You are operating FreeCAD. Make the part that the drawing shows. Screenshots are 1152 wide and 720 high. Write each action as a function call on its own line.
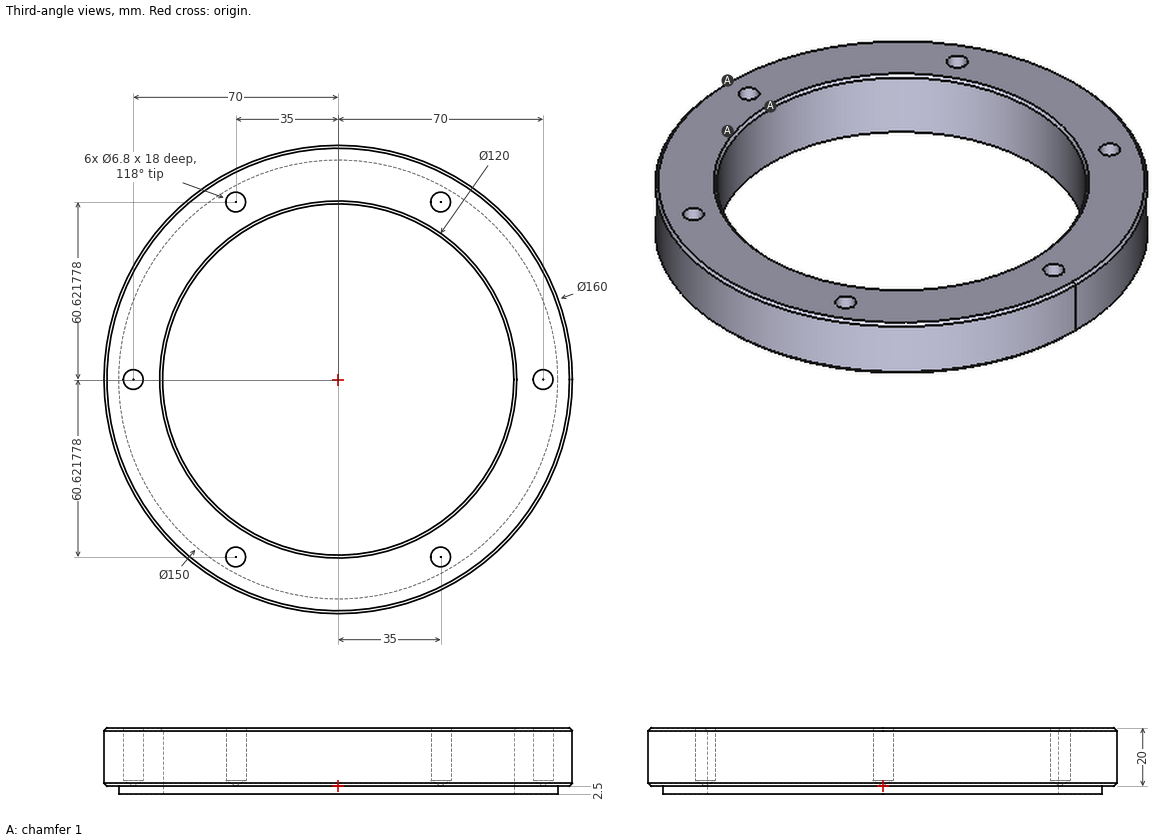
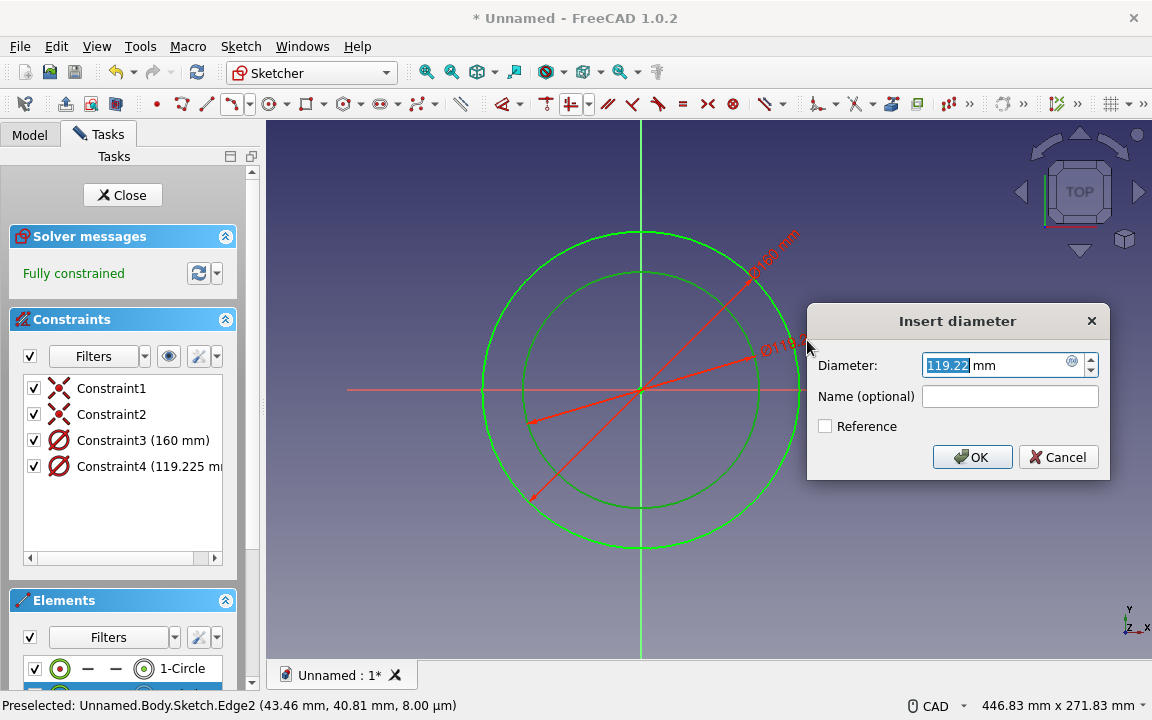
text(120)
key(Return)
key(Escape)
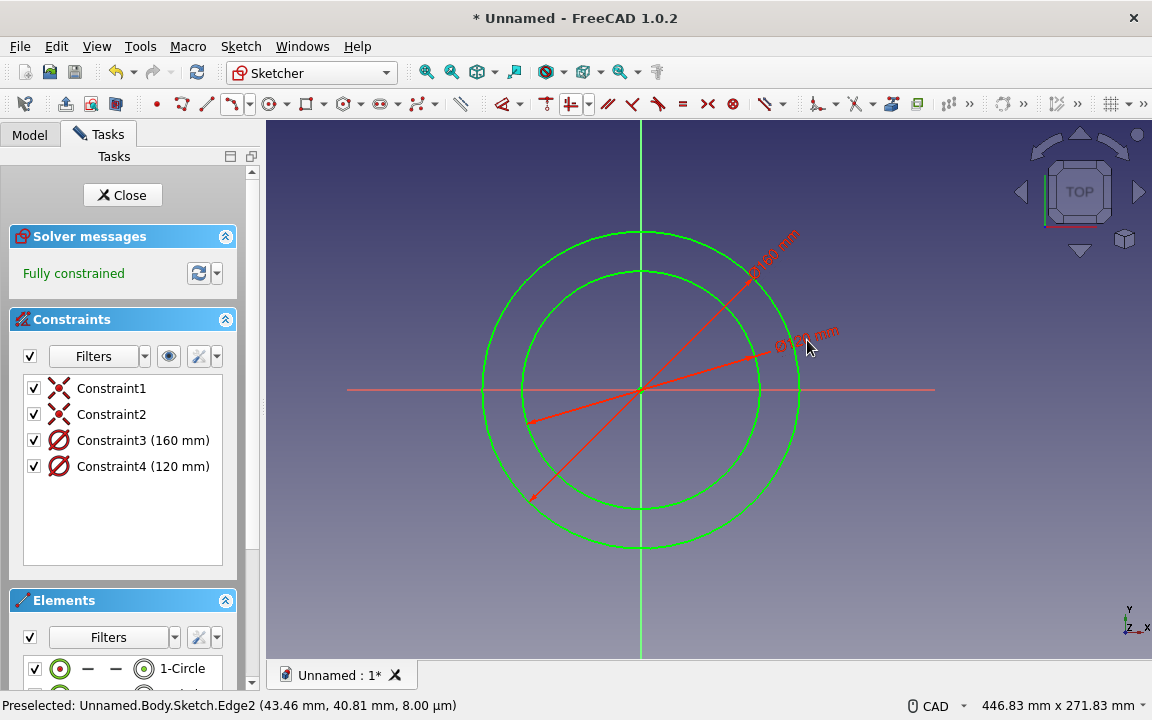
click(123, 195)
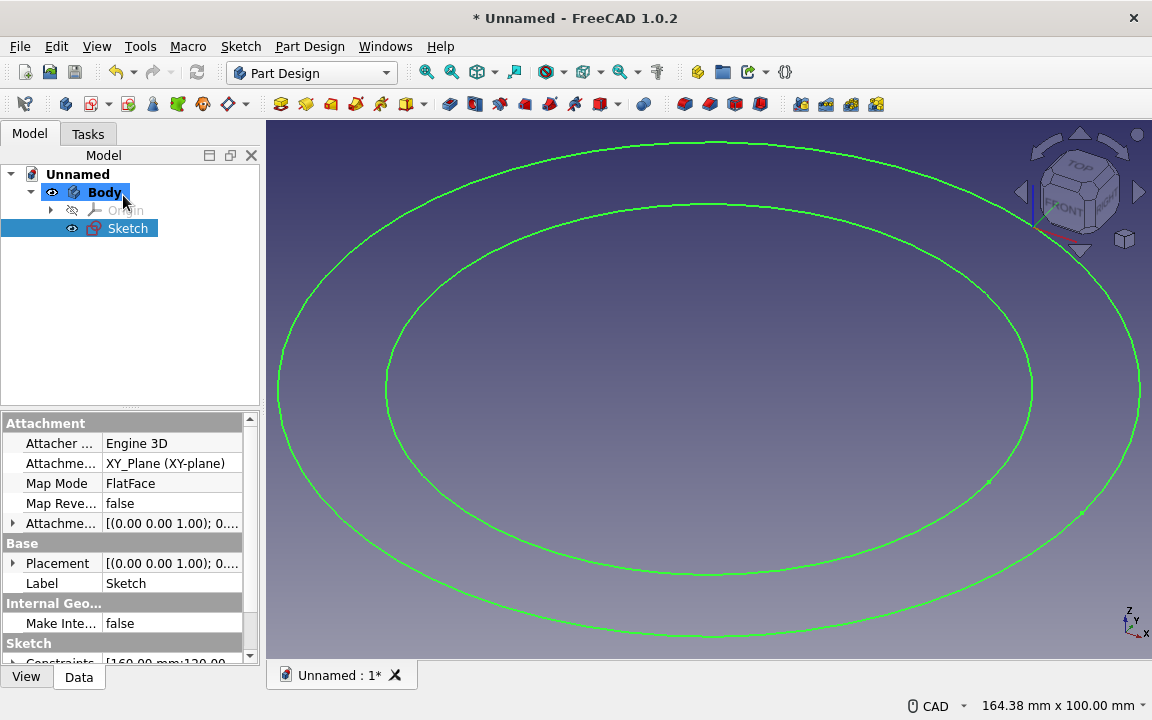
click(281, 104)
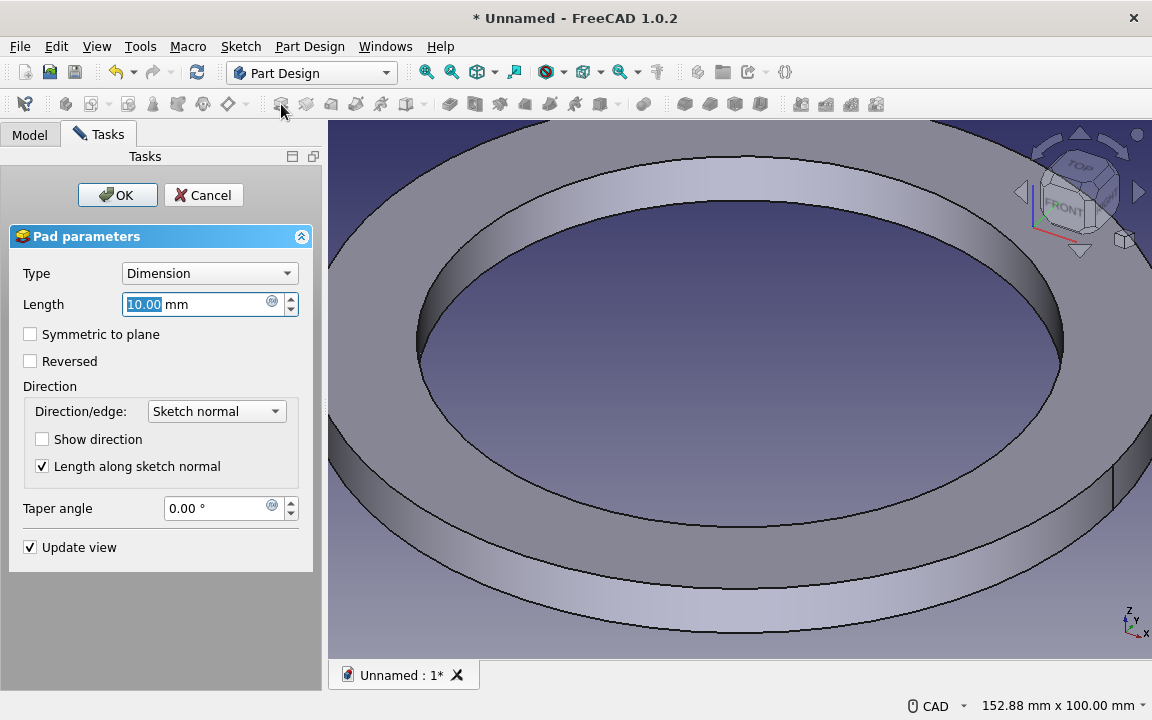
text(20)
key(Tab)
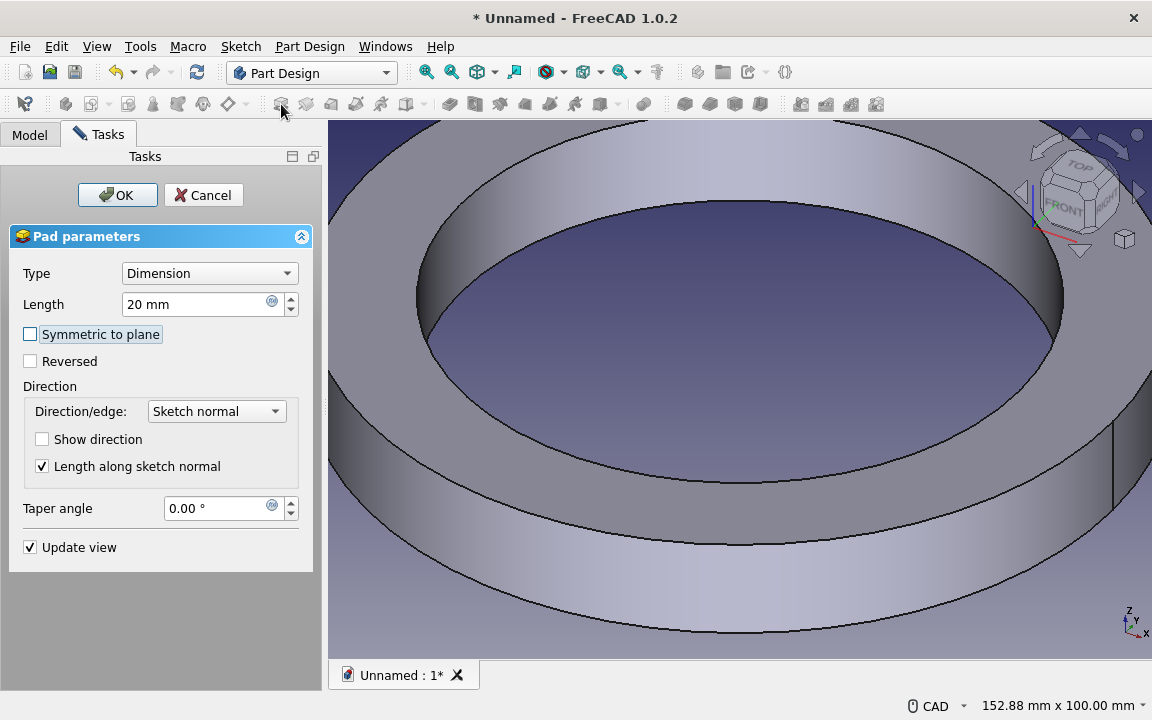
click(118, 195)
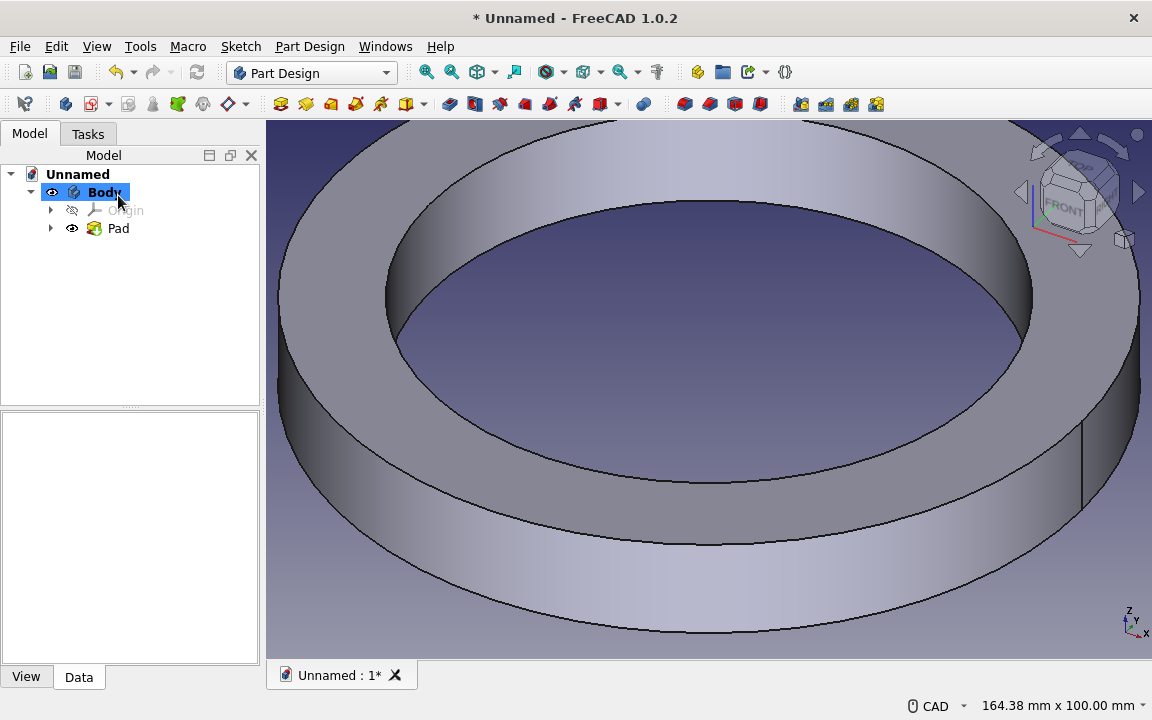
click(427, 72)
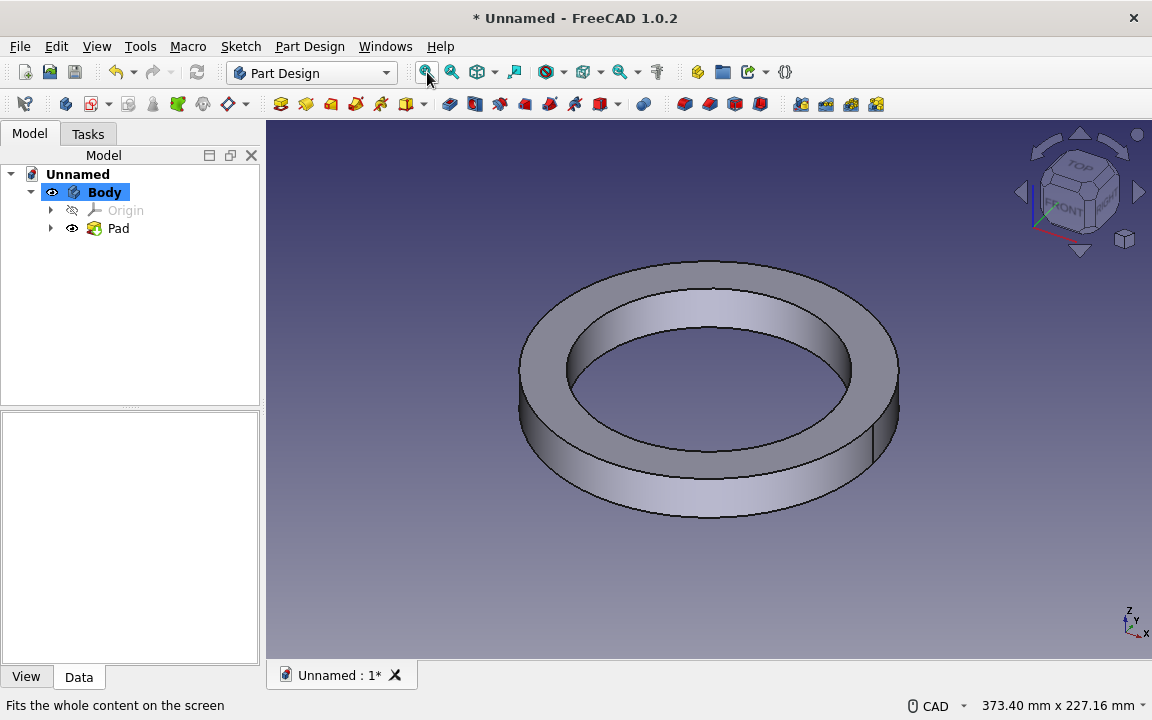
click(850, 416)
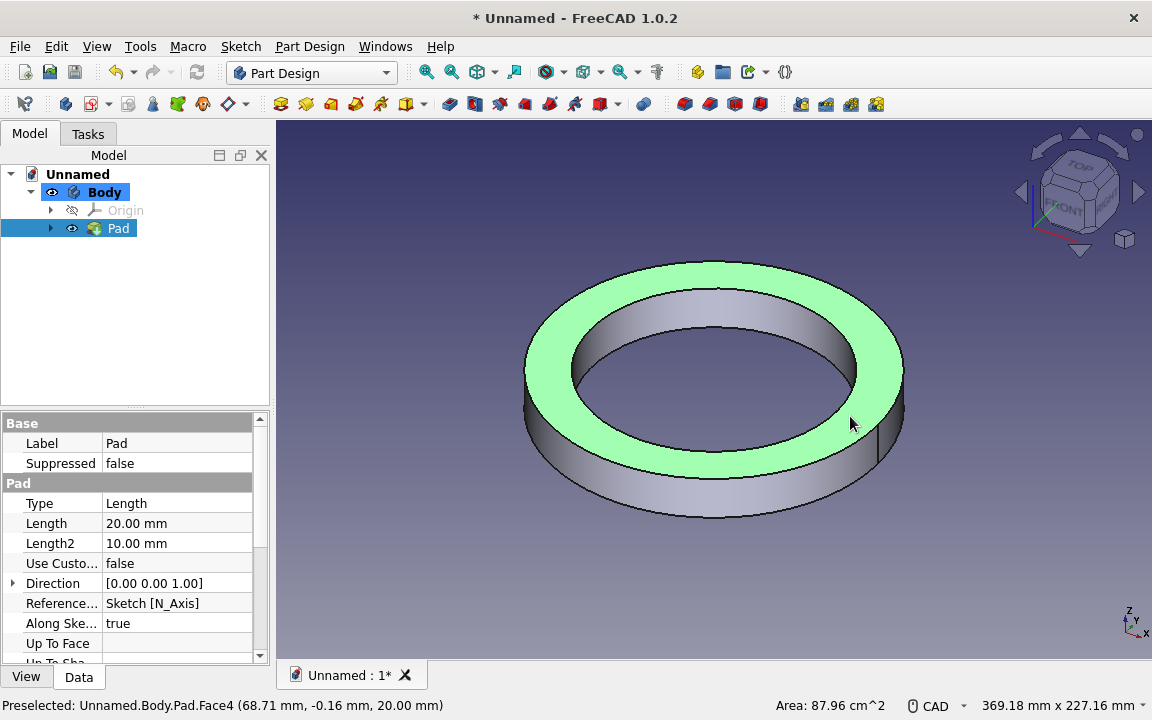
click(90, 104)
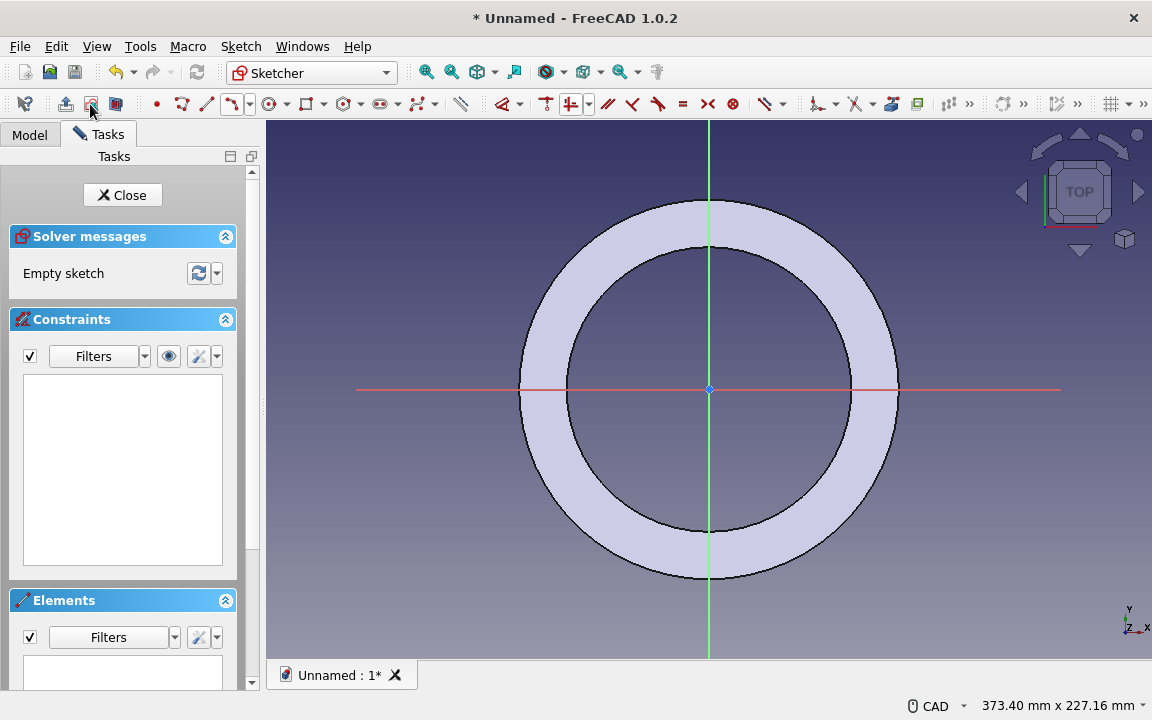
click(268, 104)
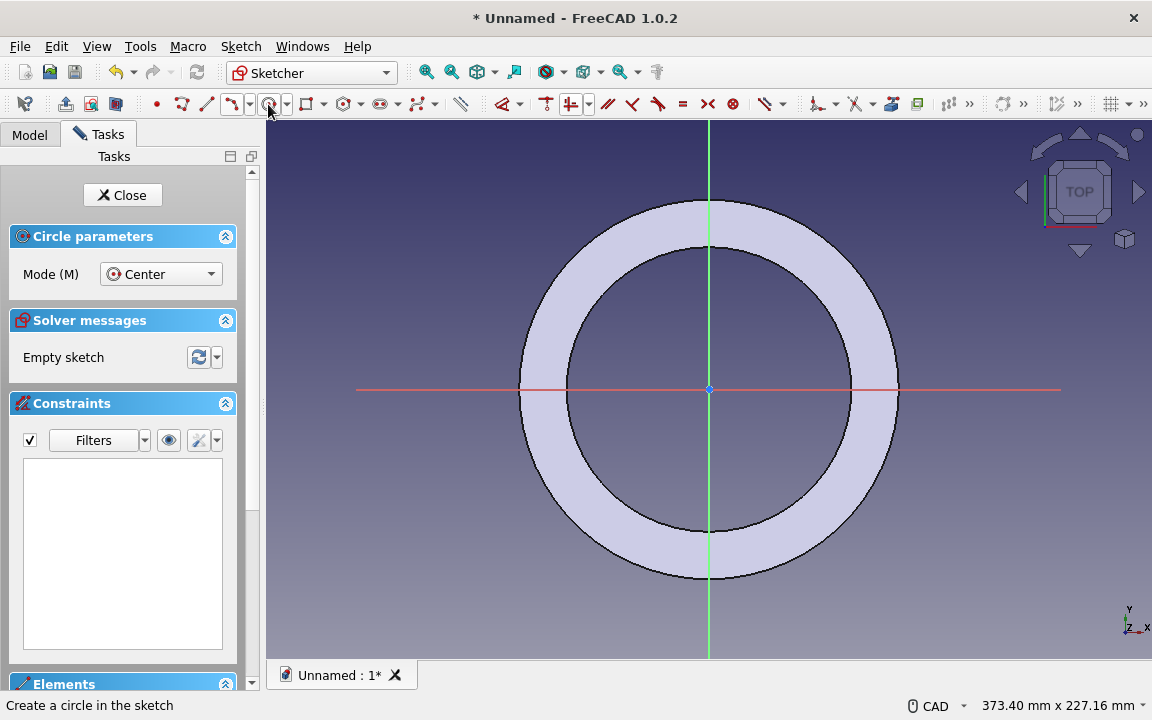
scroll(626, 246, up, 6)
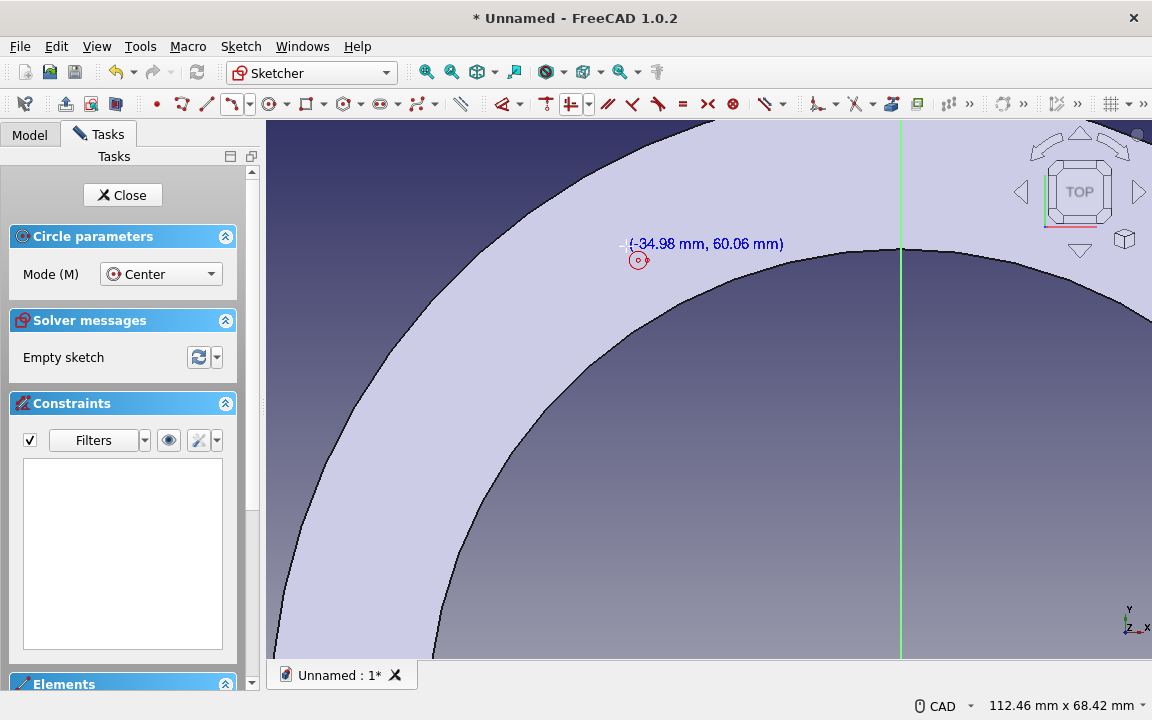
click(625, 244)
click(644, 225)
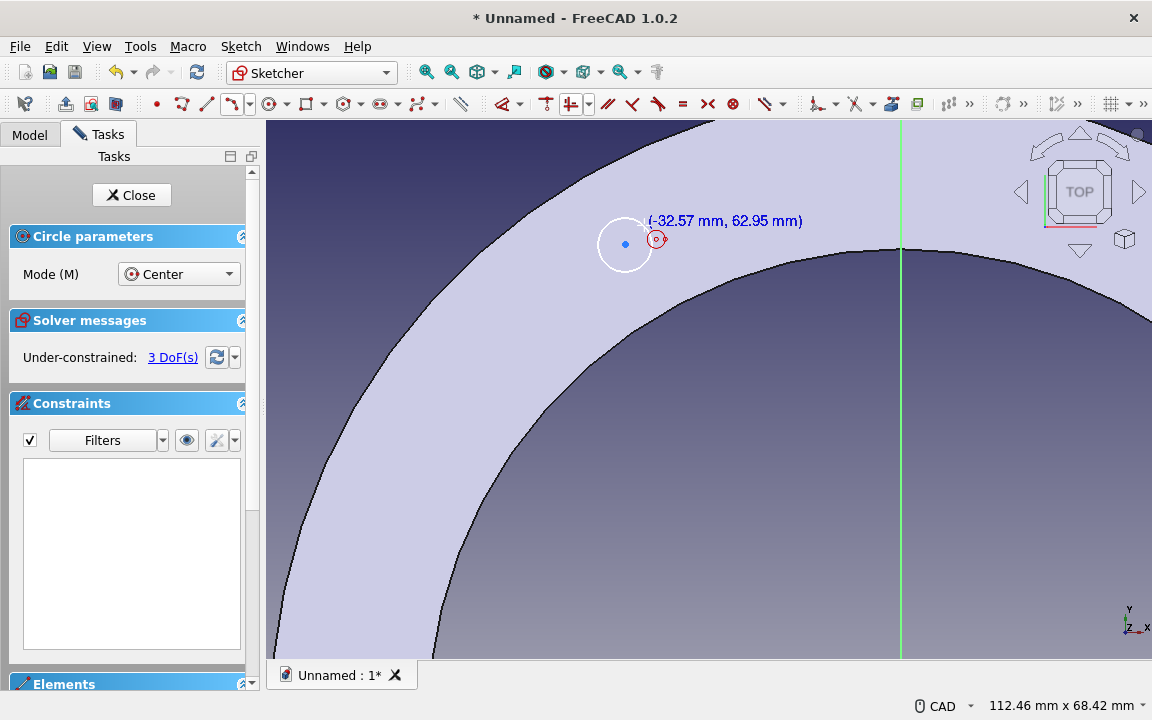
scroll(489, 196, down, 5)